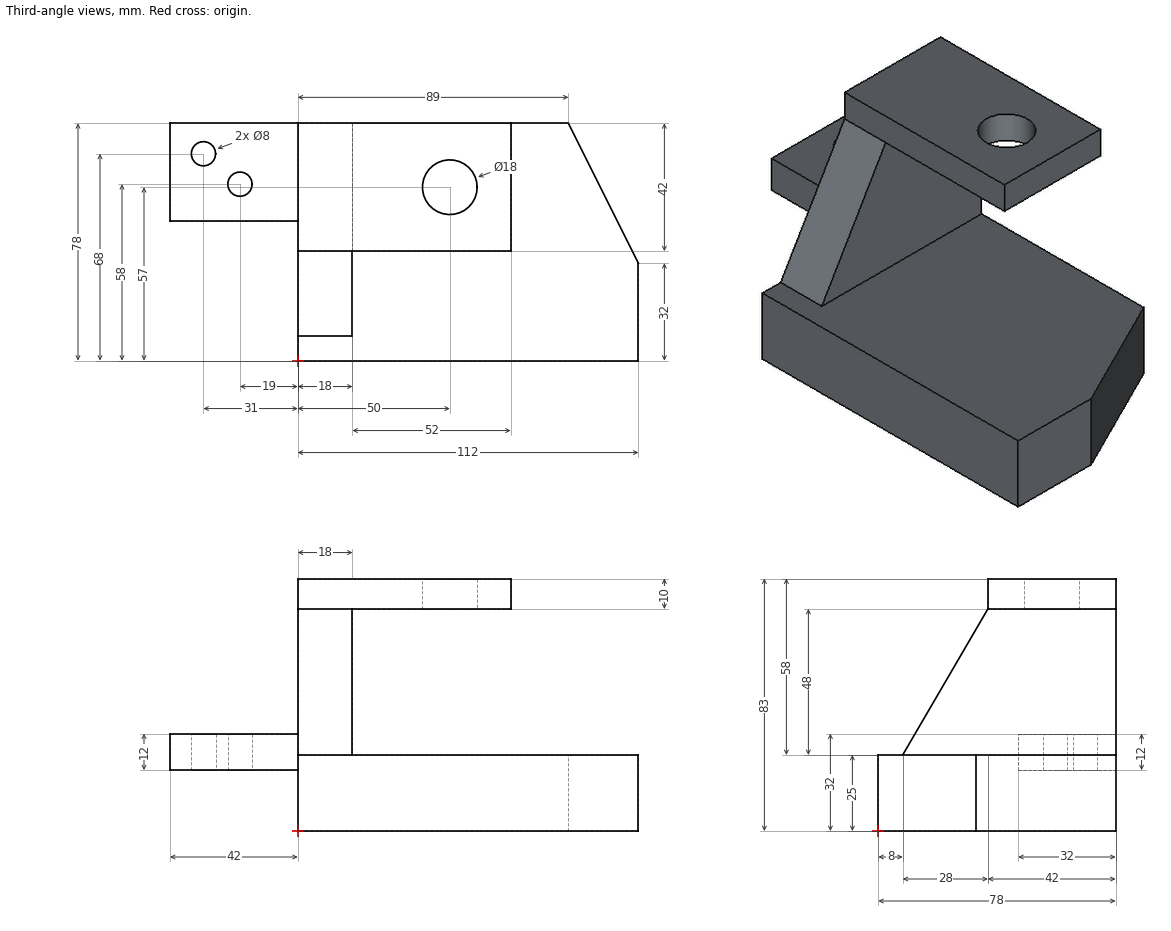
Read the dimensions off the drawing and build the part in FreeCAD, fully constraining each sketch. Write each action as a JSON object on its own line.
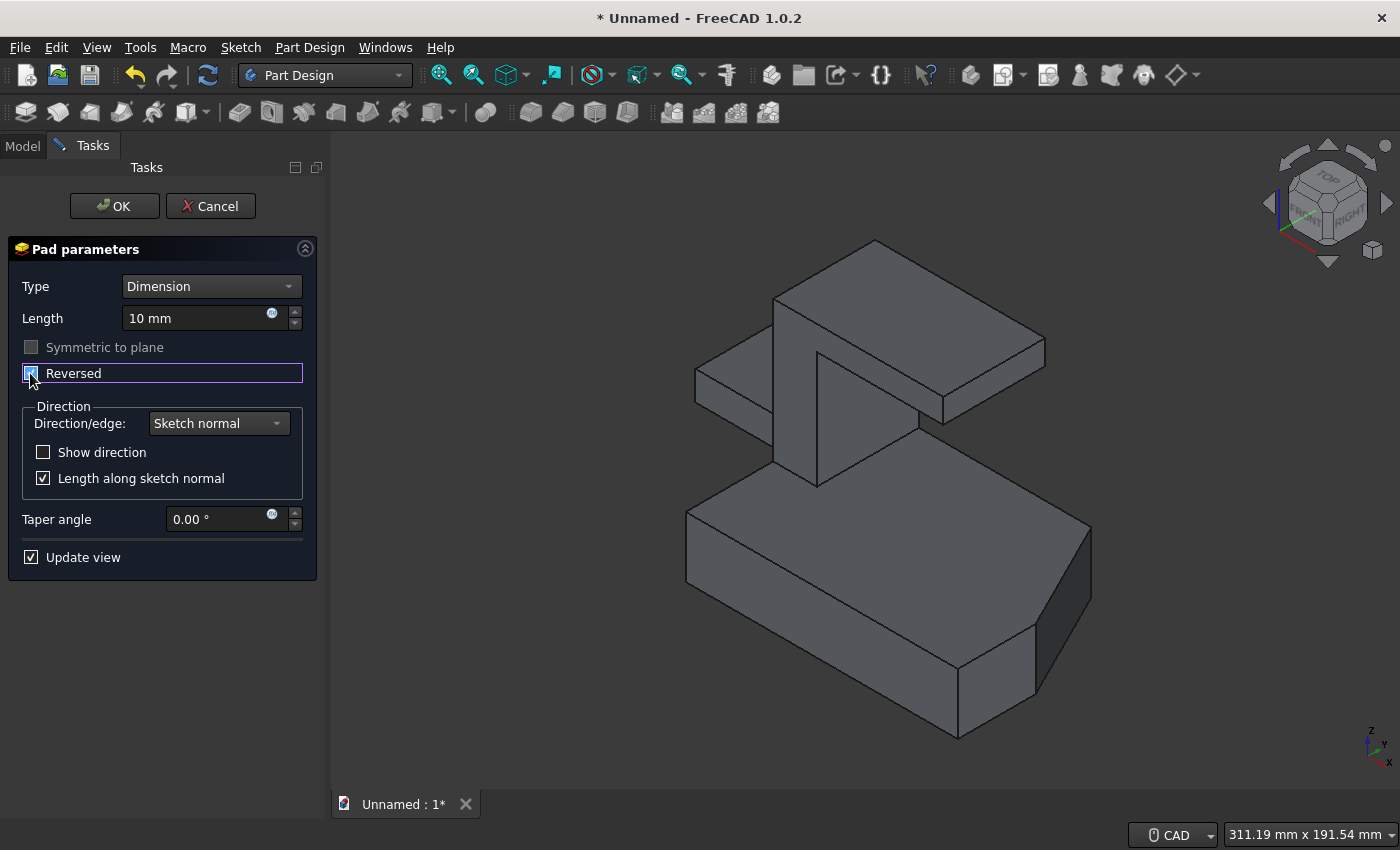
{"action": "left_click", "coordinate": [115, 206]}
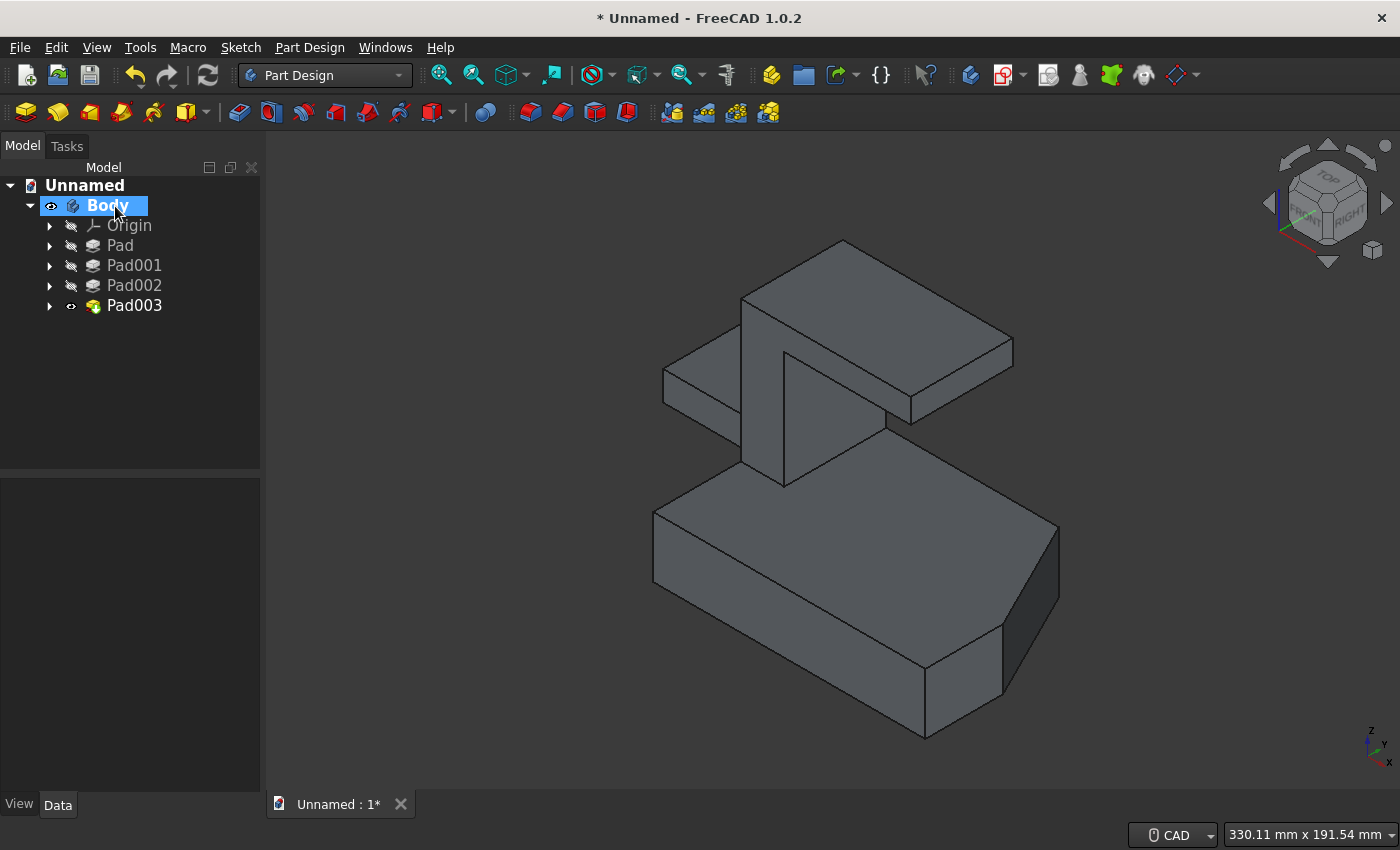
{"action": "left_click", "coordinate": [901, 331]}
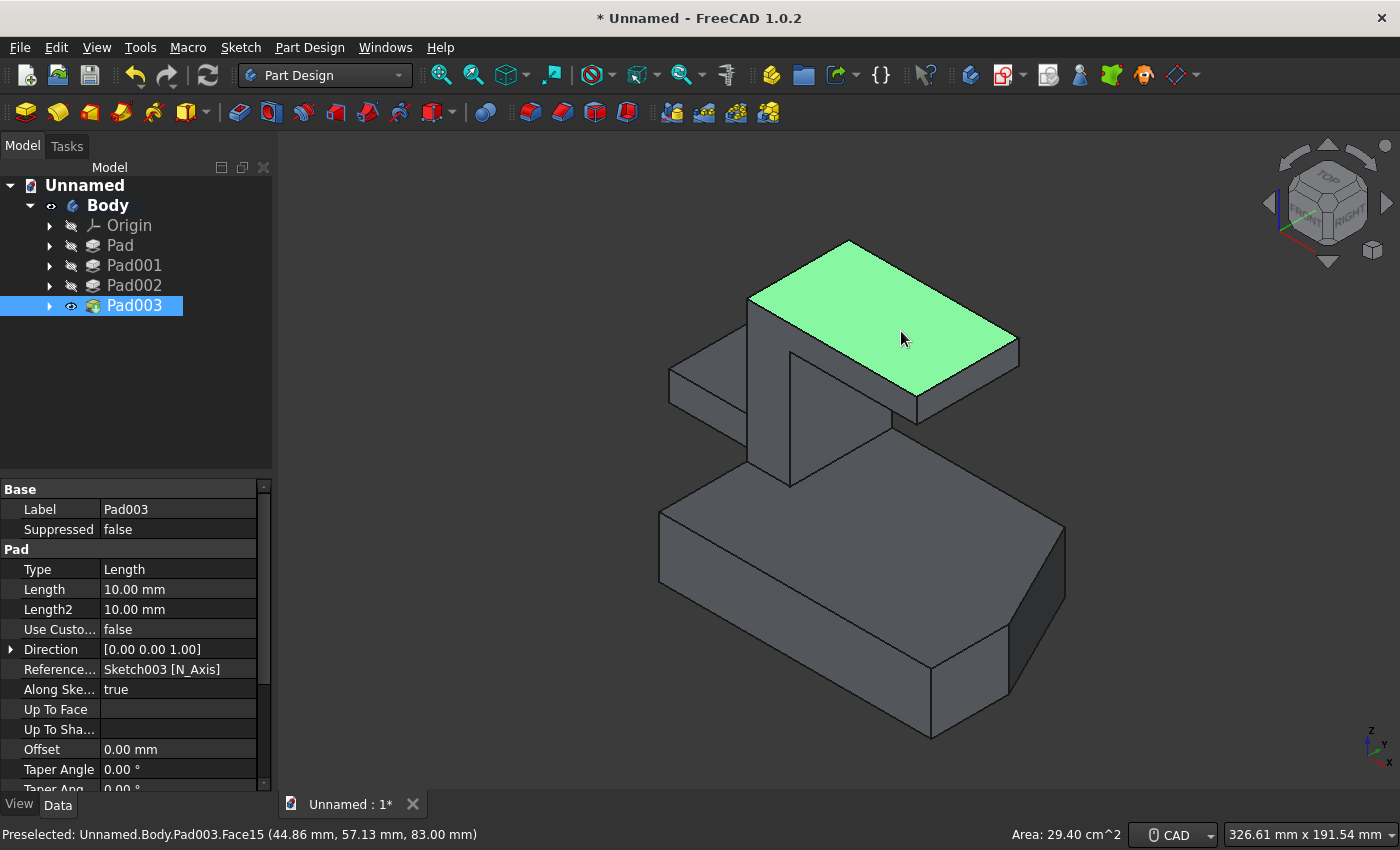
{"action": "left_click", "coordinate": [1004, 76]}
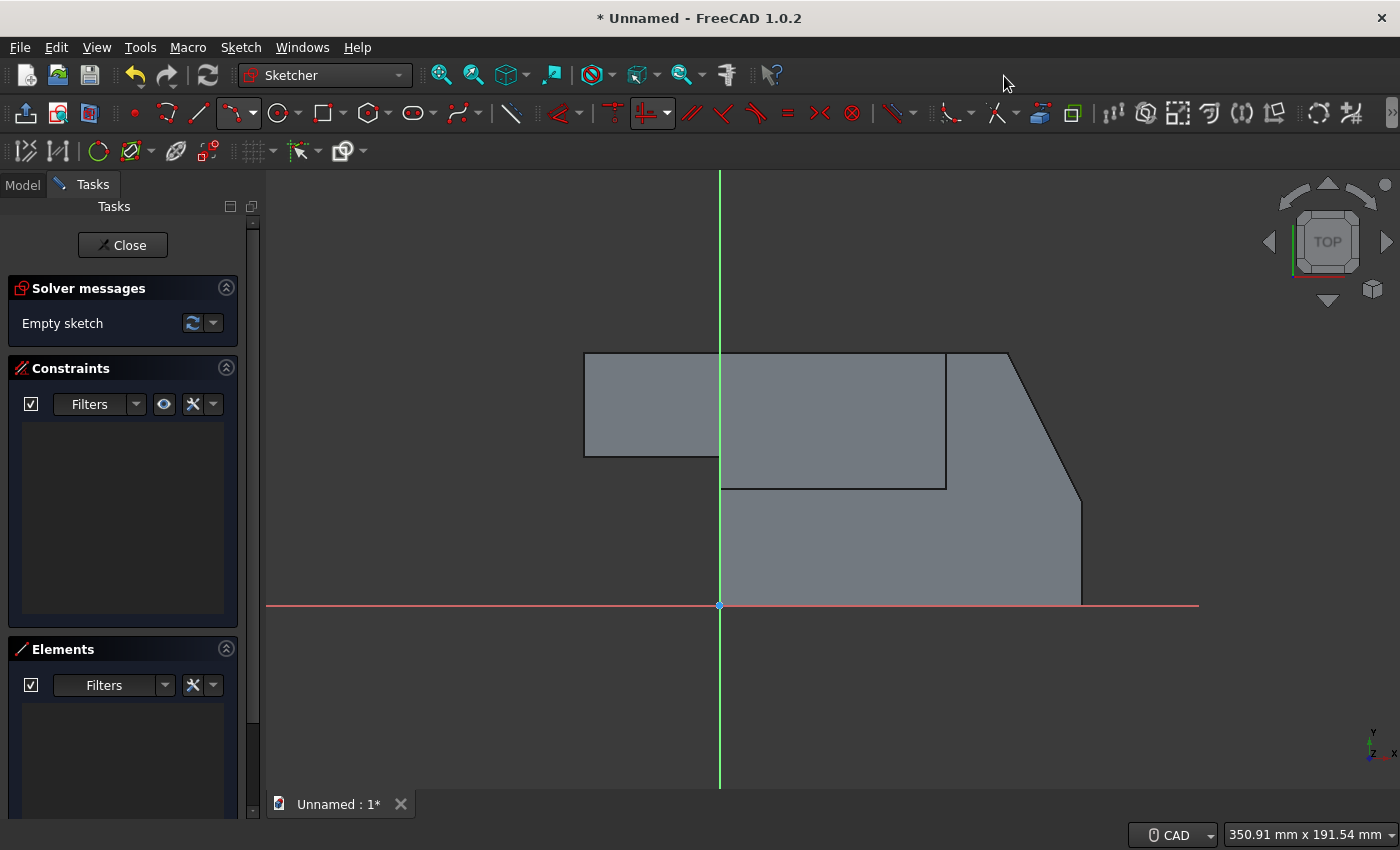
{"action": "scroll", "coordinate": [900, 412], "scroll_direction": "up", "scroll_amount": 10}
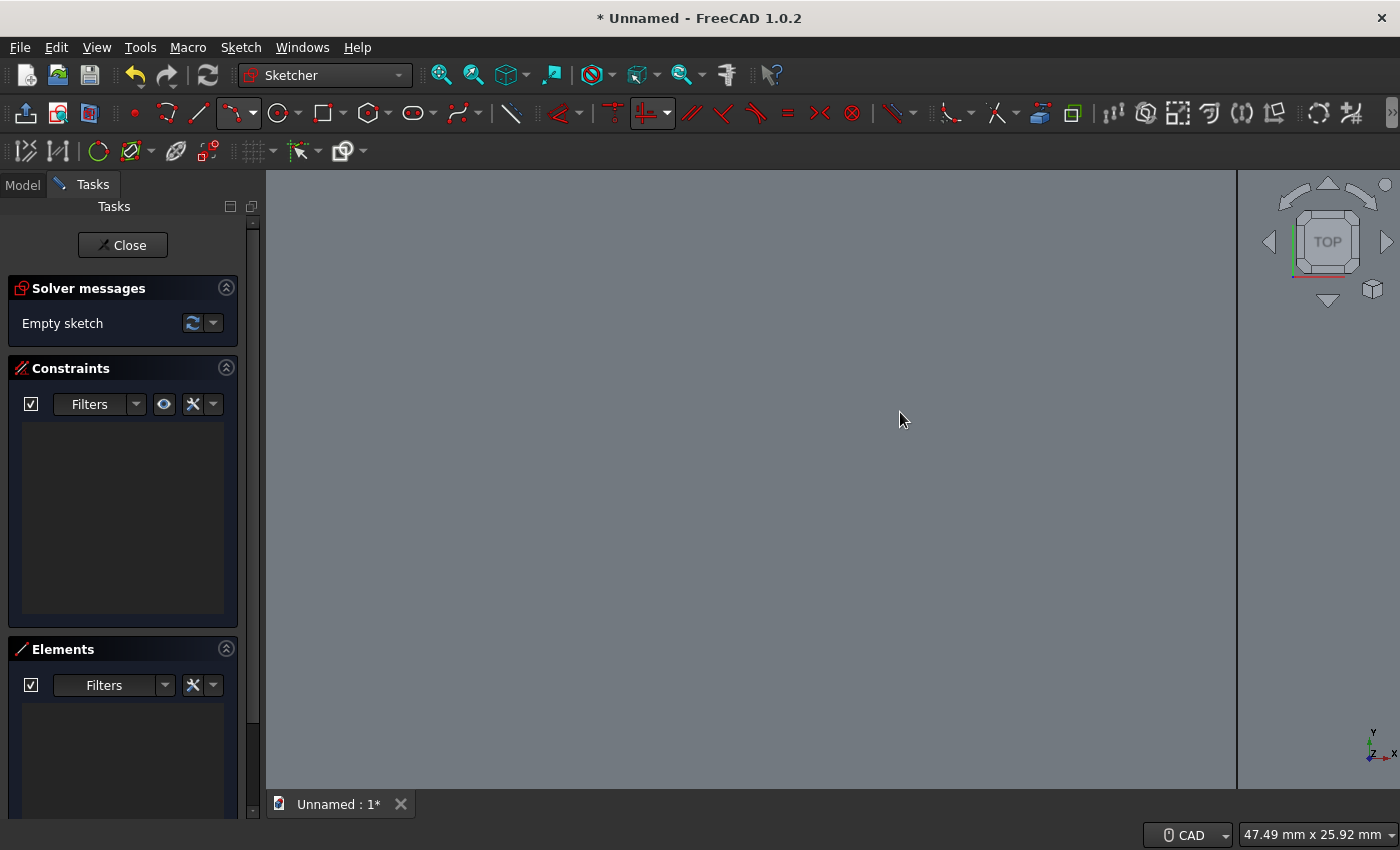
{"action": "left_click", "coordinate": [278, 114]}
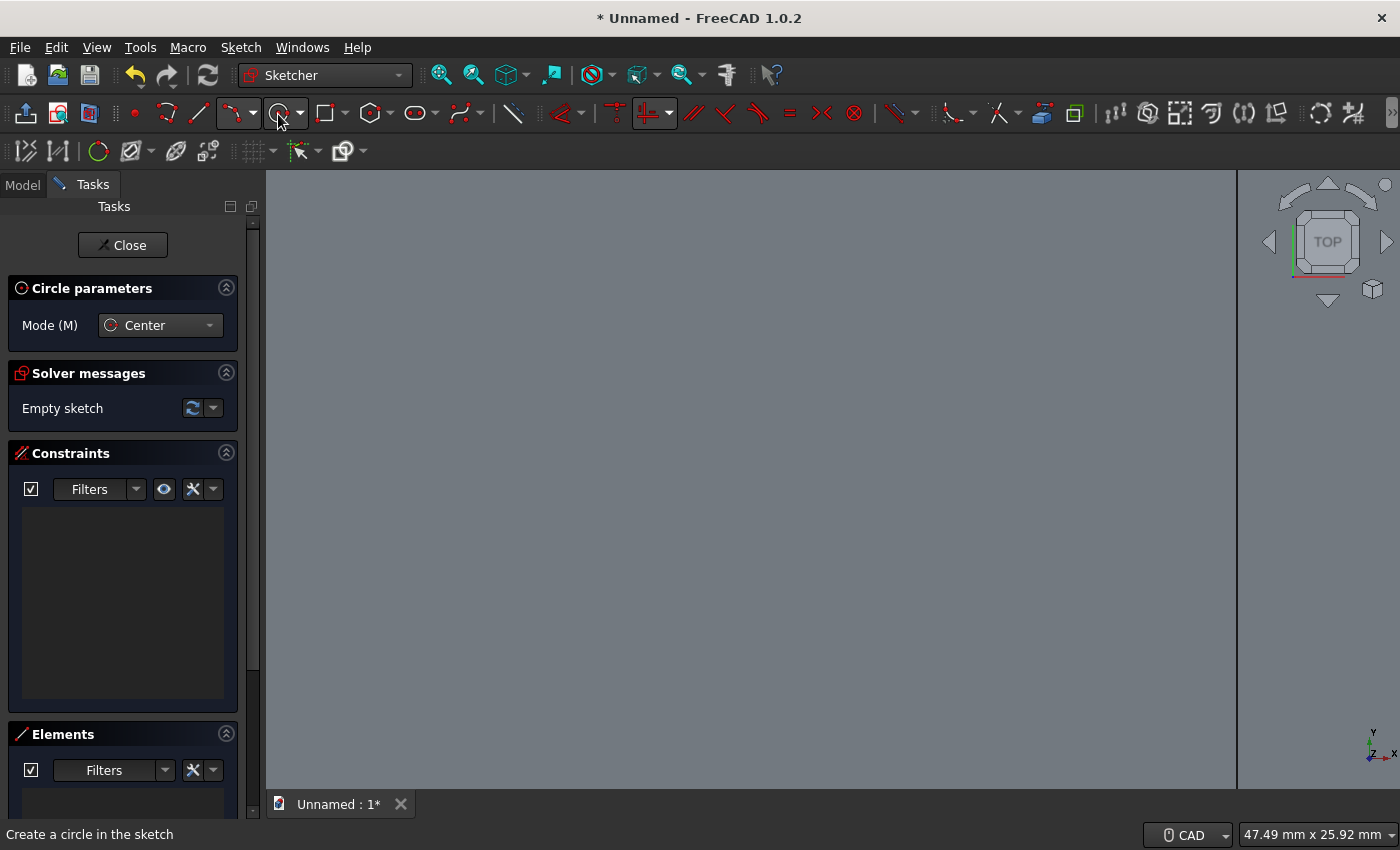
{"action": "left_click", "coordinate": [760, 478]}
{"action": "mouse_move", "coordinate": [912, 326]}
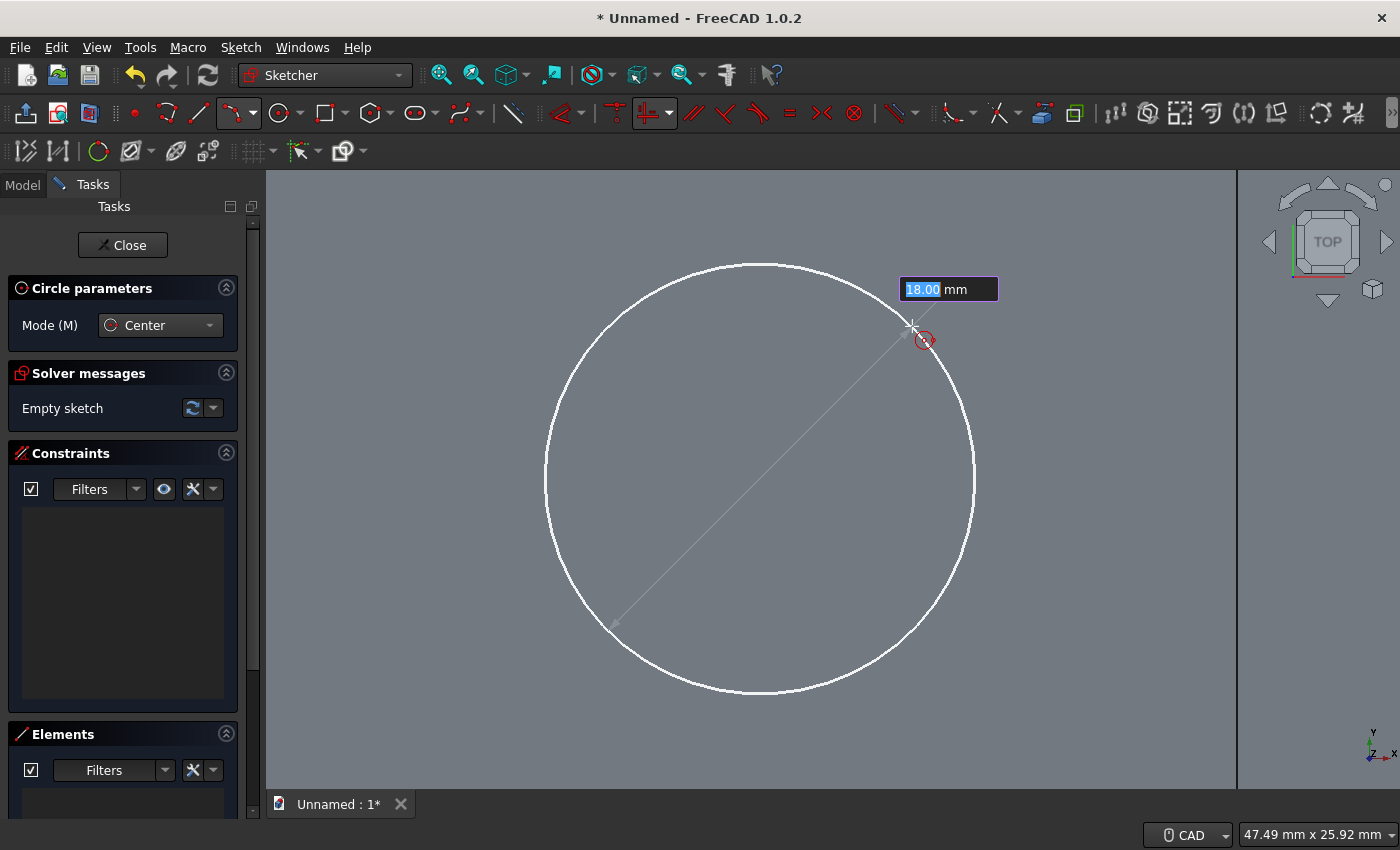
{"action": "type", "text": "18"}
{"action": "key", "text": "Return"}
{"action": "key", "text": "Escape"}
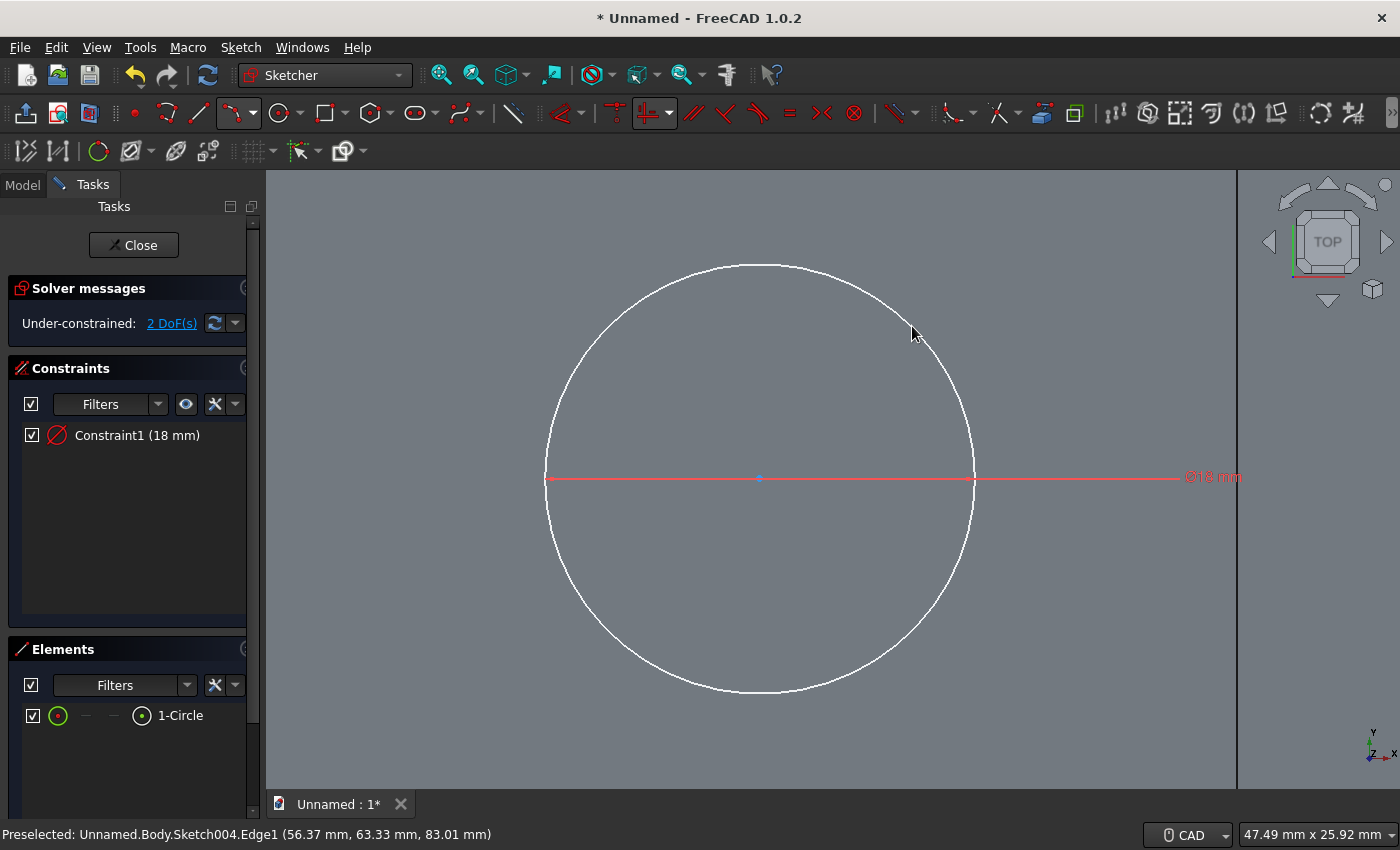
{"action": "key", "text": "d"}